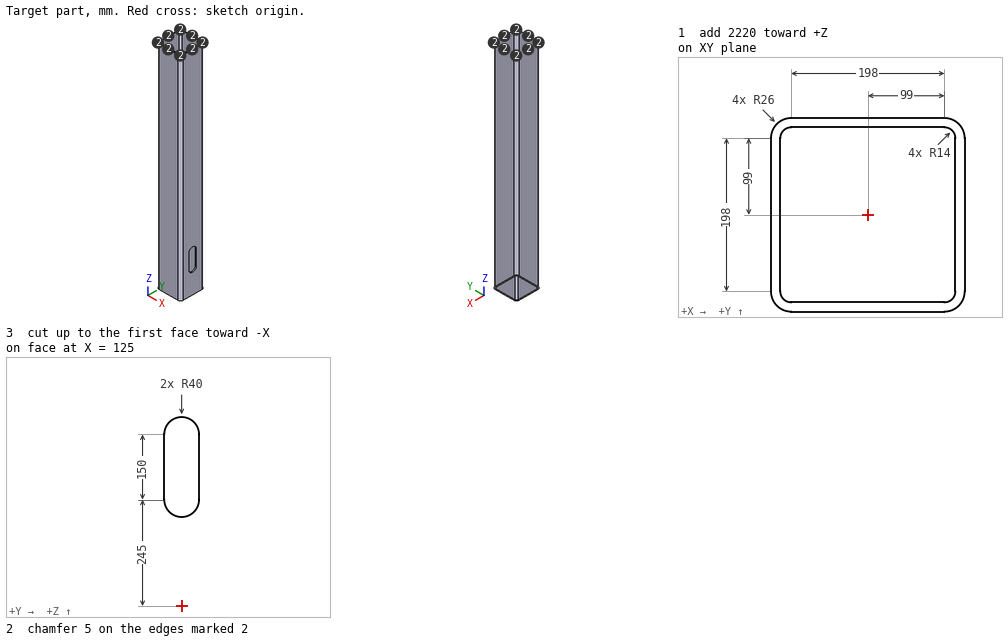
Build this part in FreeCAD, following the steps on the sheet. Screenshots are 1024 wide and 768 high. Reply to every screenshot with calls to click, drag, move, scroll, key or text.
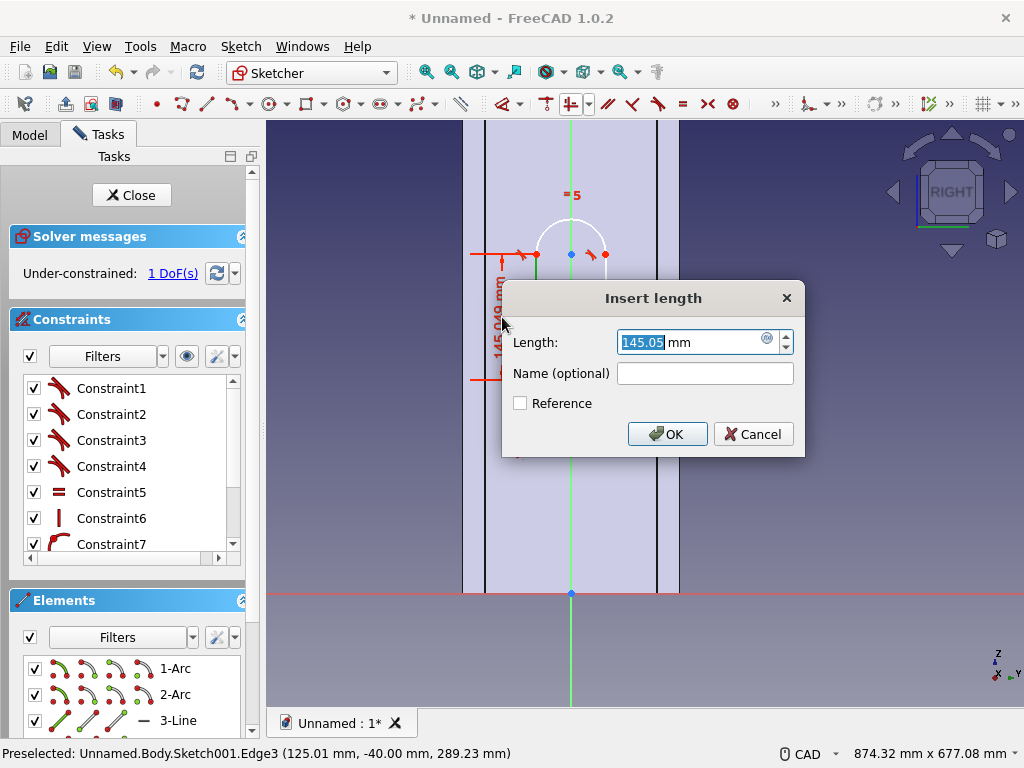
text(150)
key(Return)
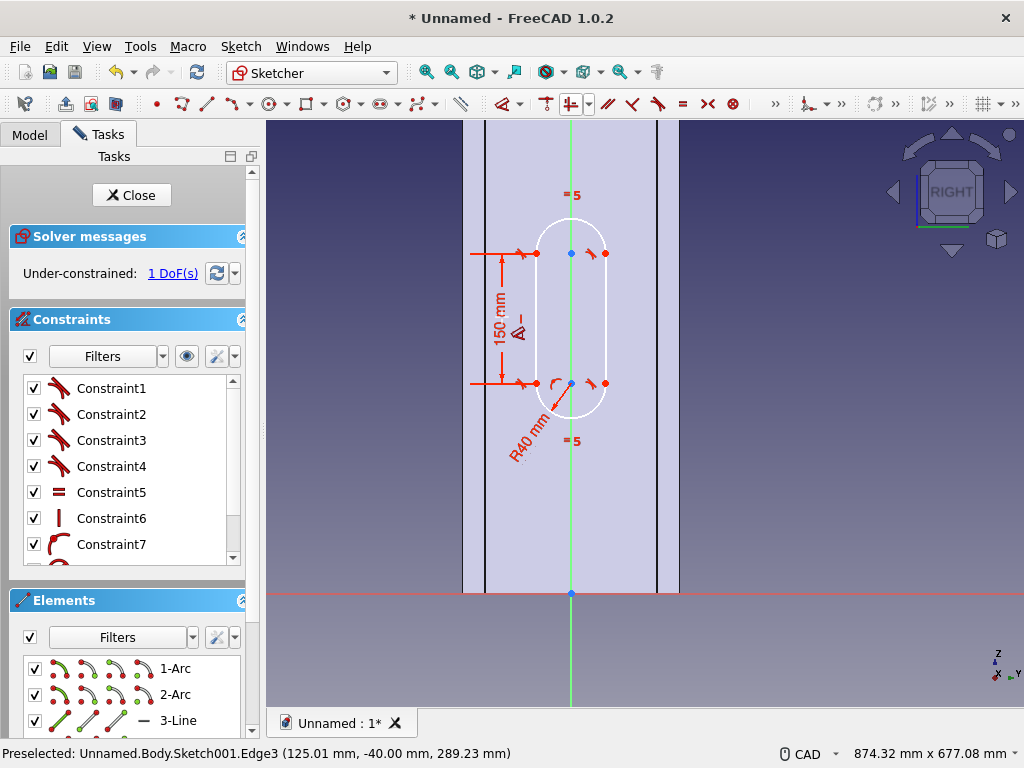
click(536, 384)
click(502, 489)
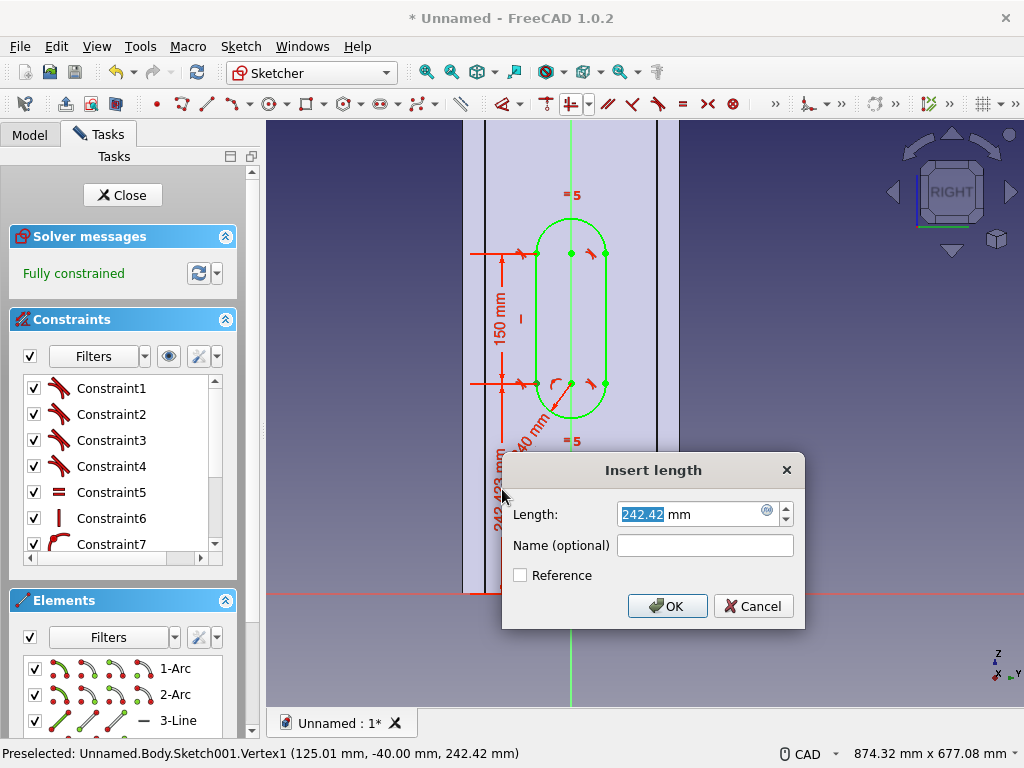
text(245)
key(Return)
key(Escape)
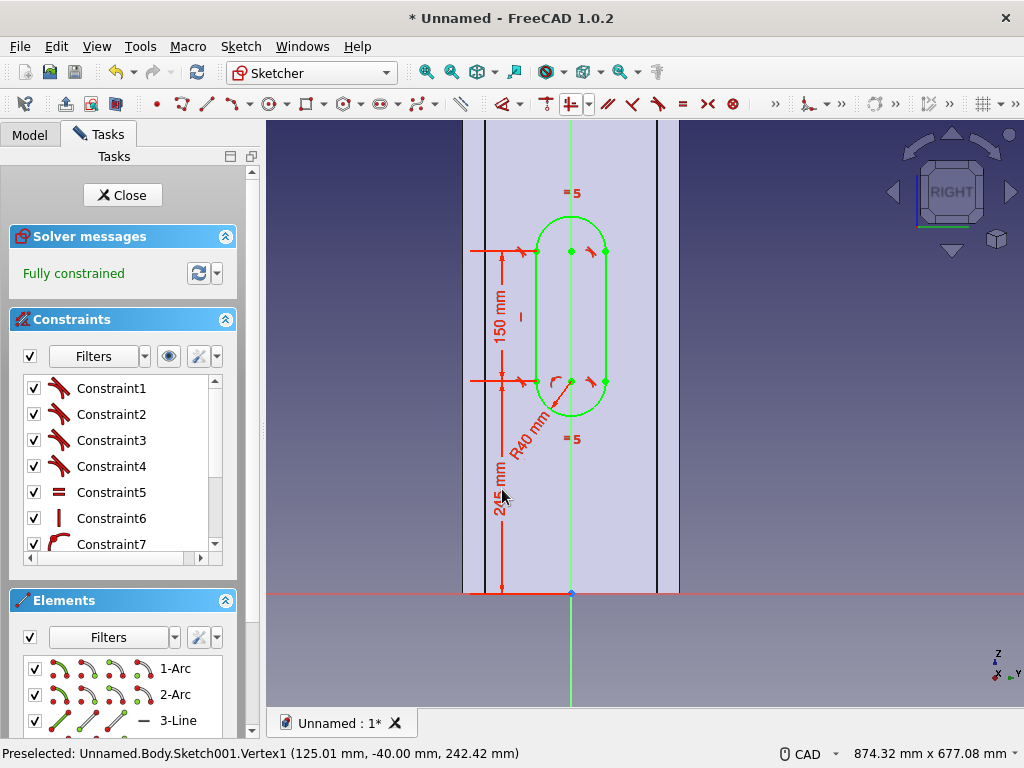
click(123, 195)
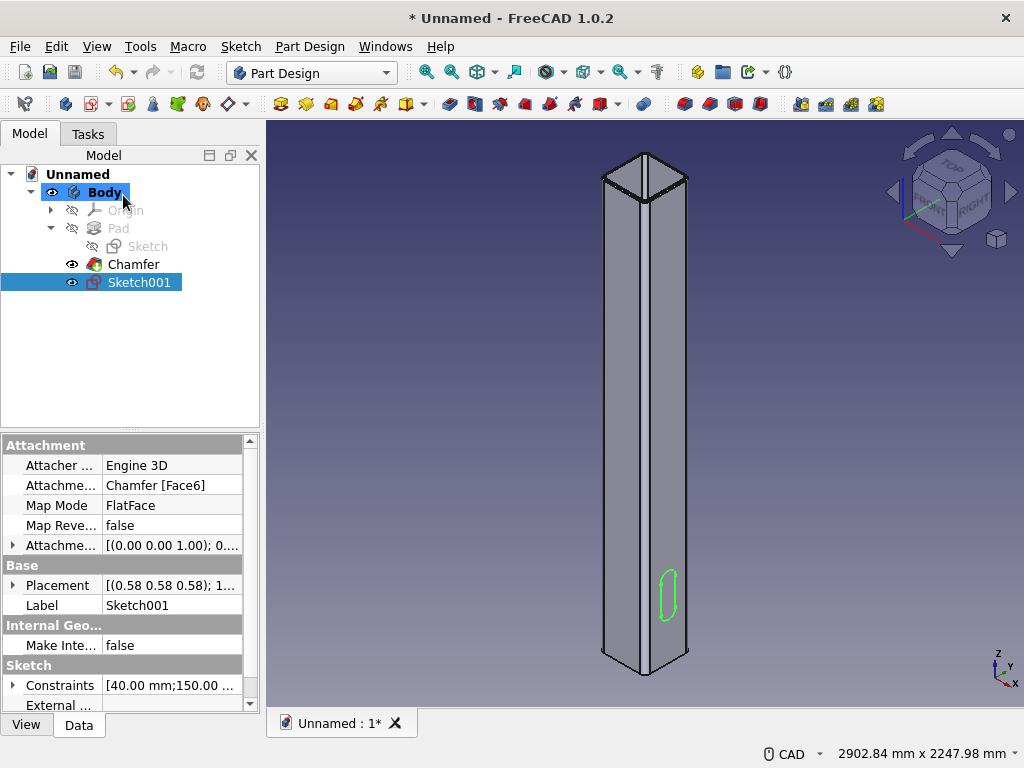
click(450, 104)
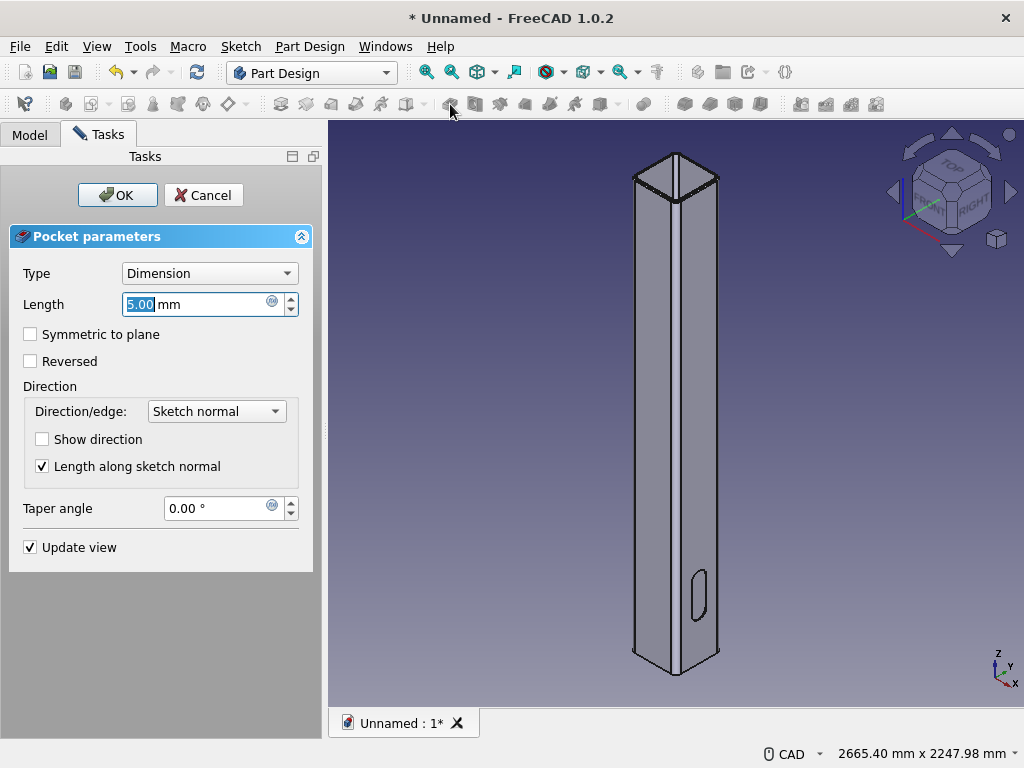
click(210, 274)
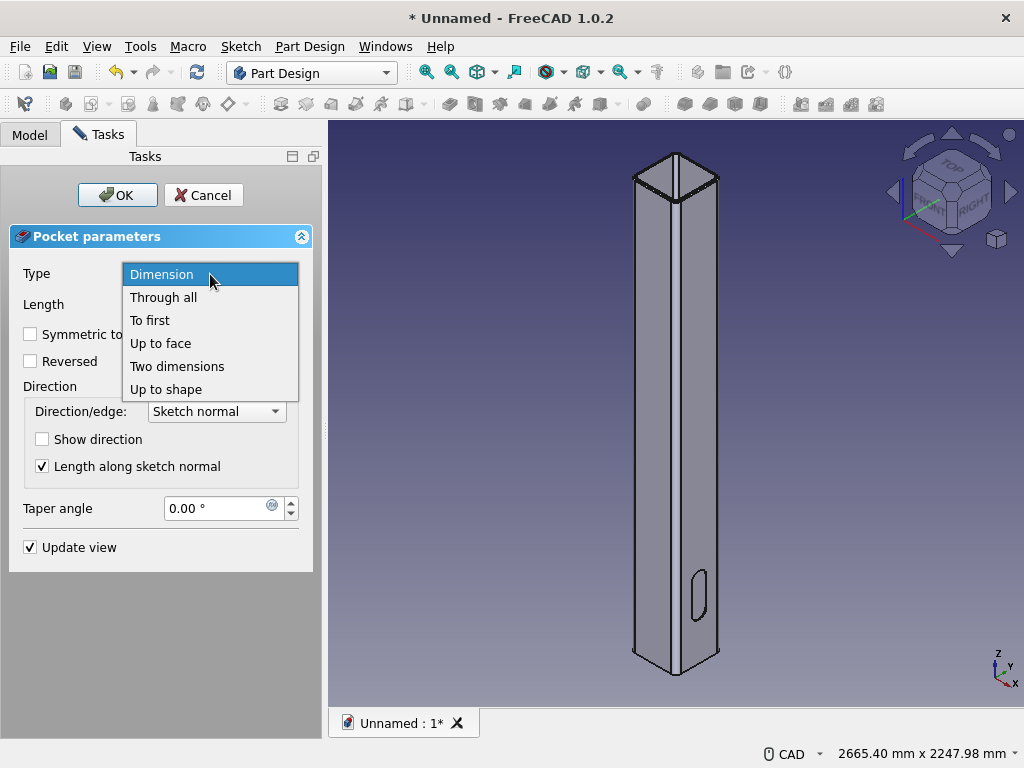
click(208, 320)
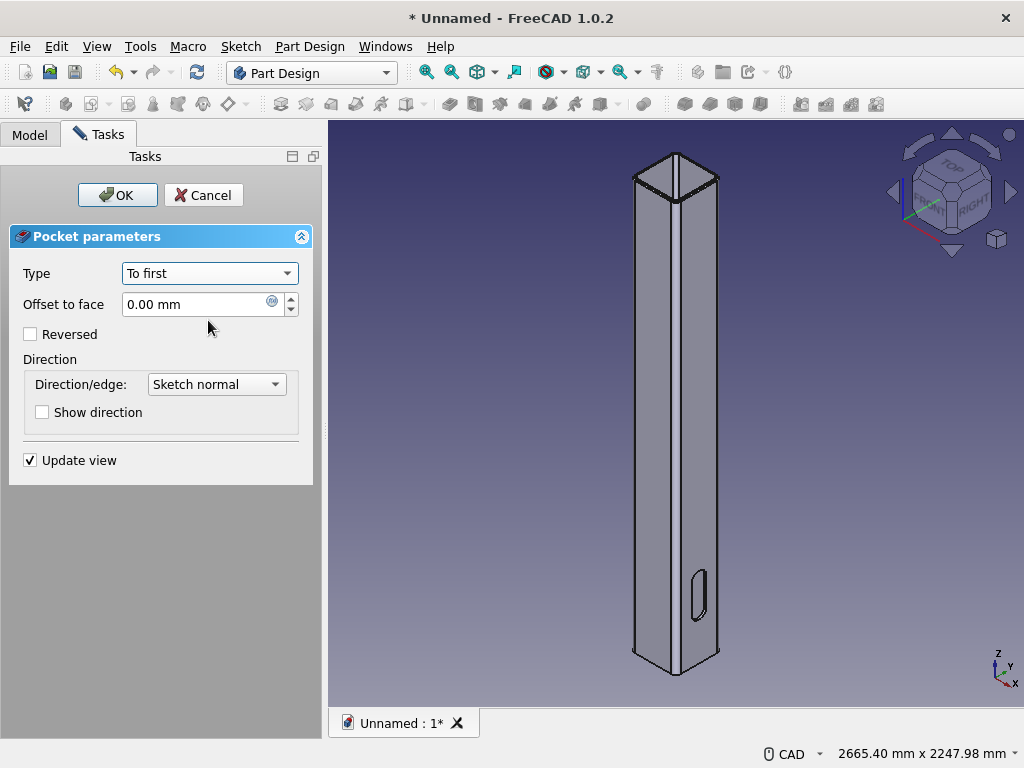
click(118, 195)